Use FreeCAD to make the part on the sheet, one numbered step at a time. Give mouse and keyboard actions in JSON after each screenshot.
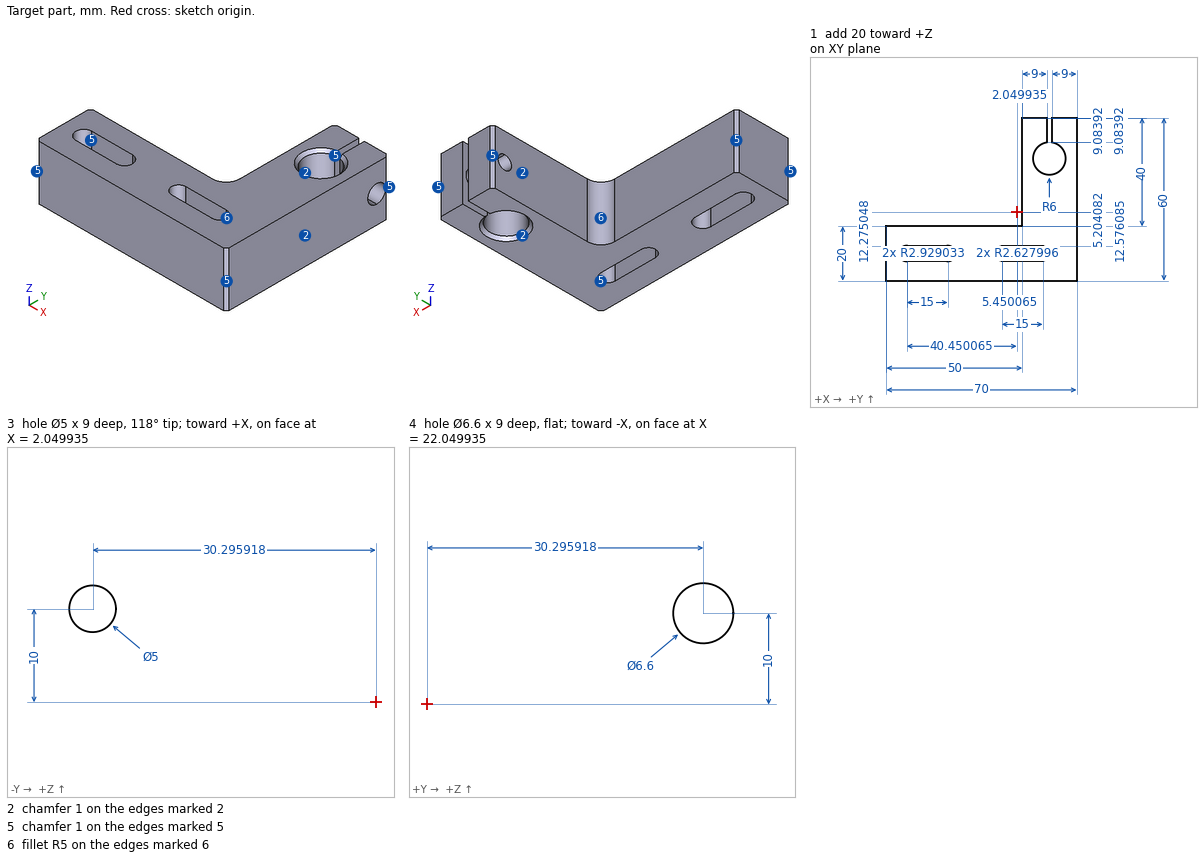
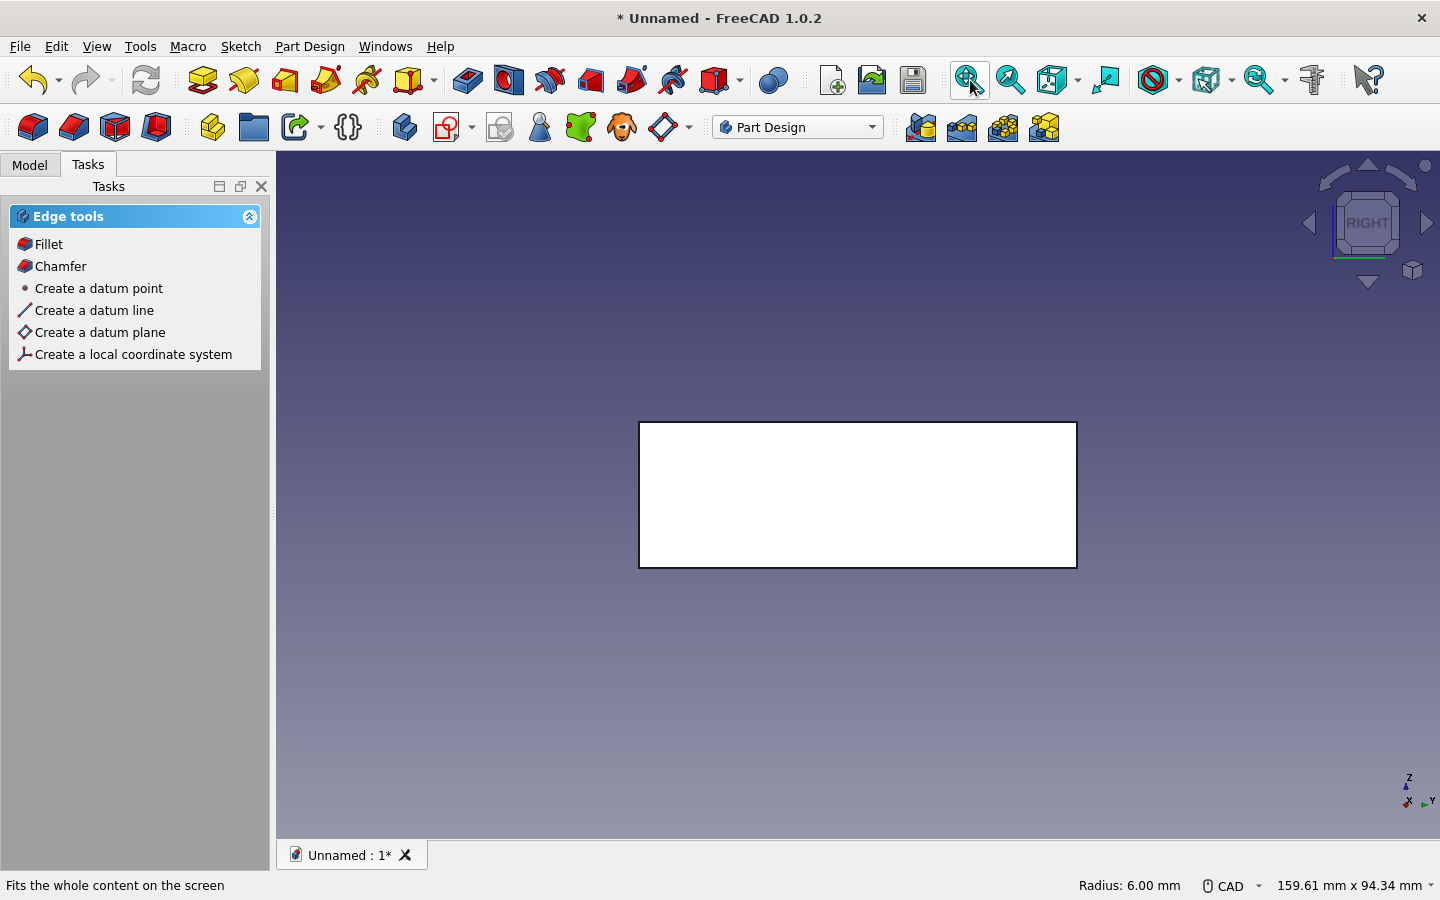
{"action": "key", "text": "5"}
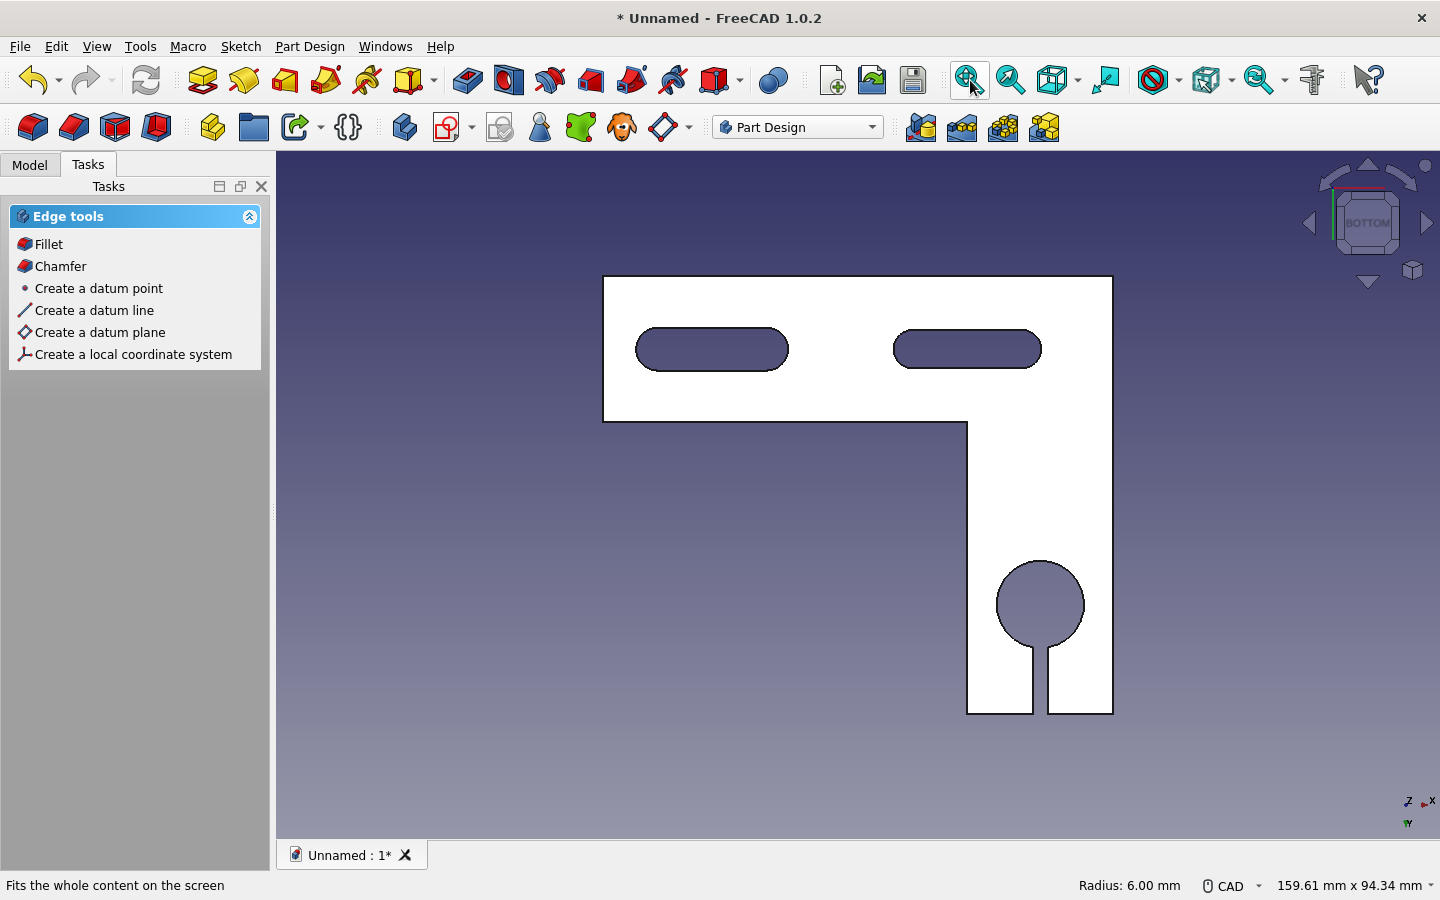
{"action": "left_click", "coordinate": [1016, 567], "text": "ctrl"}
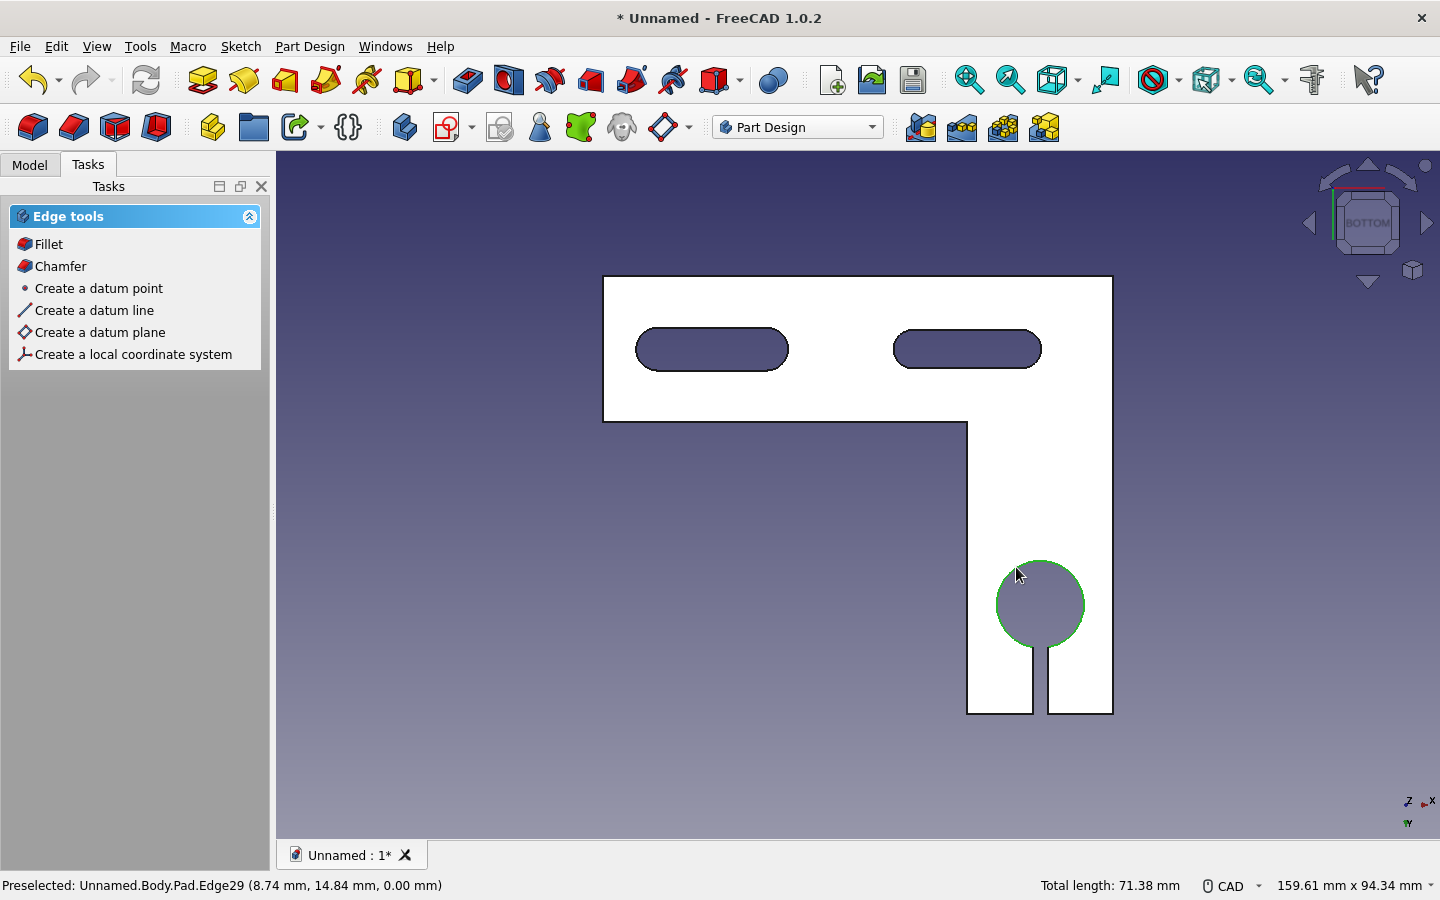
{"action": "left_click", "coordinate": [74, 128]}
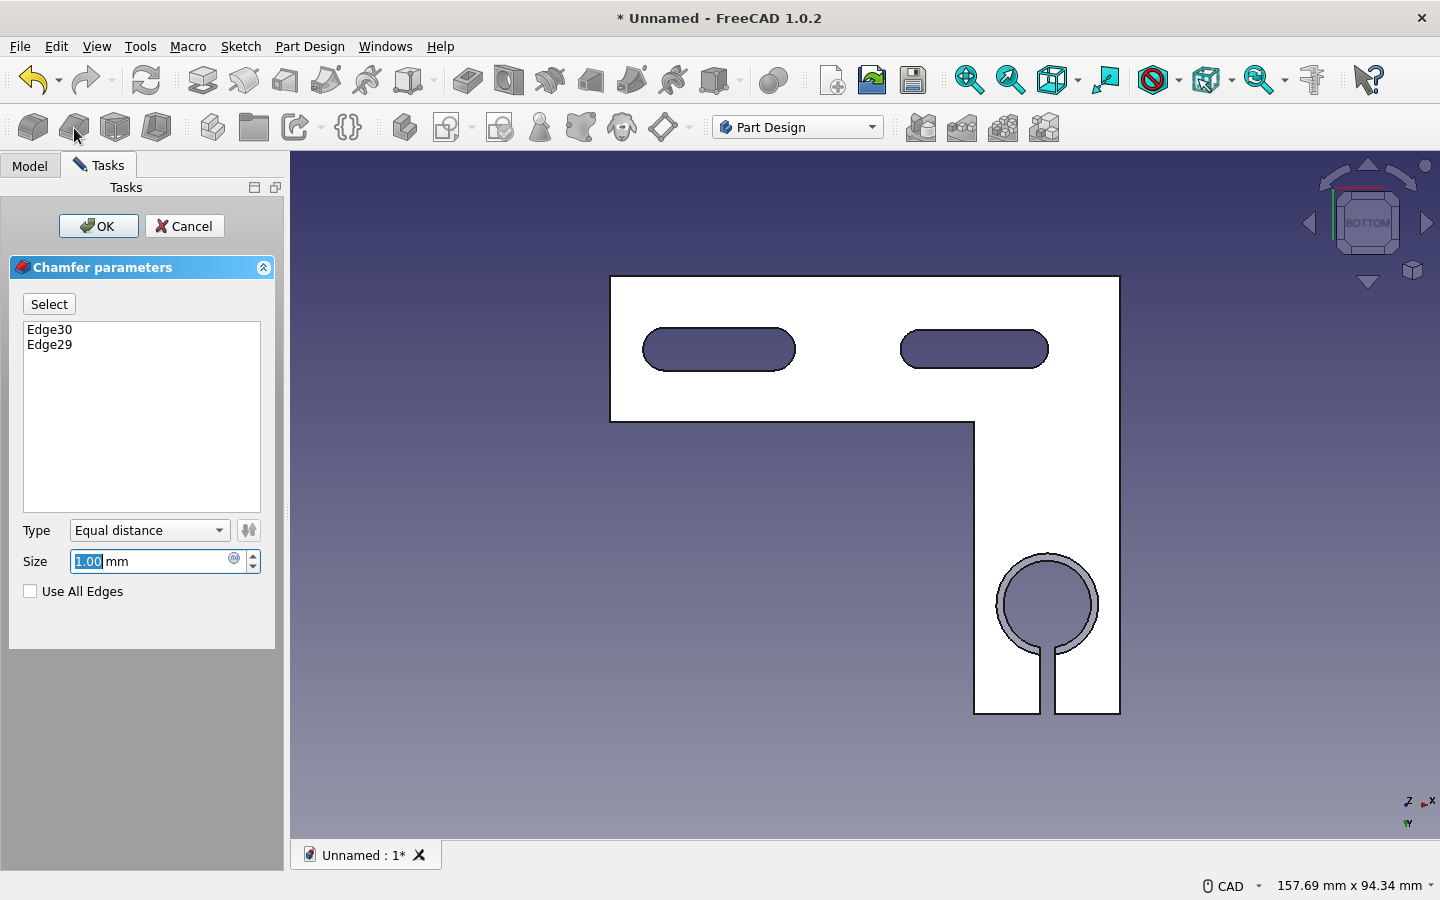
{"action": "type", "text": "1"}
{"action": "key", "text": "Tab"}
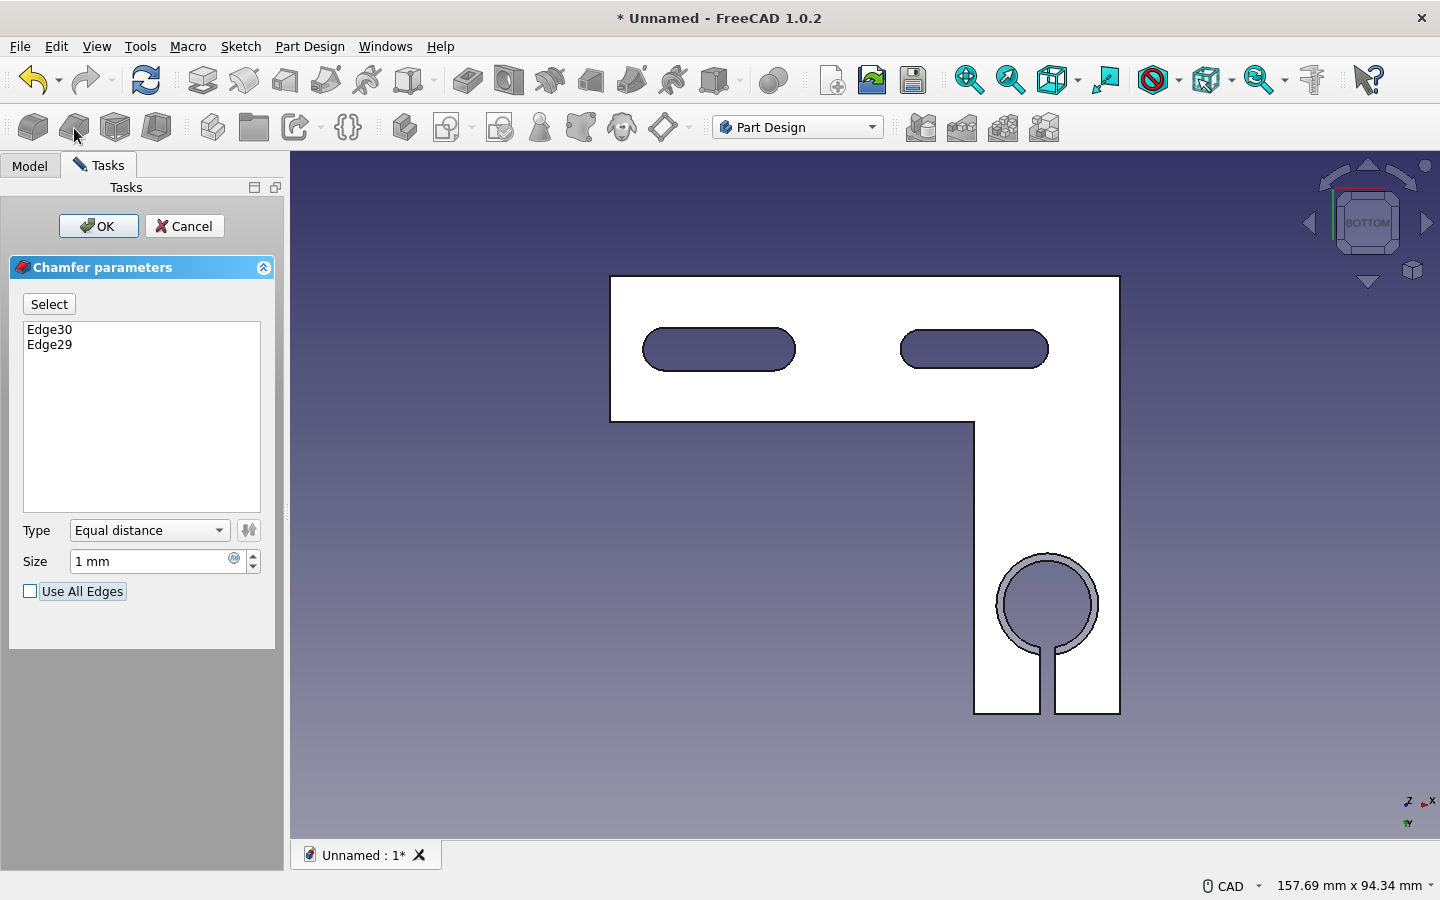
{"action": "left_click", "coordinate": [99, 226]}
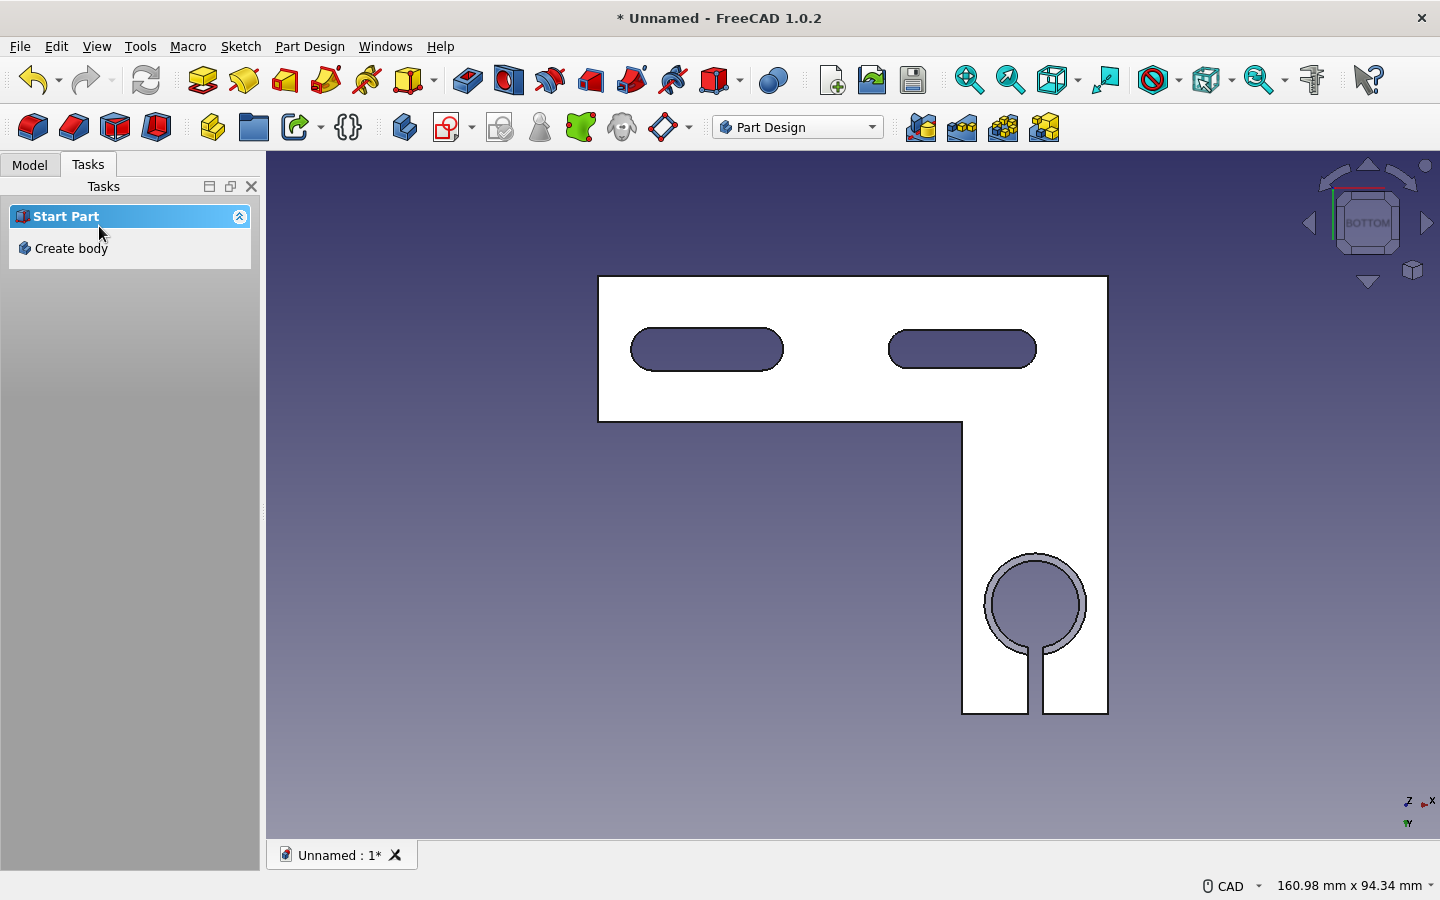
{"action": "key", "text": "6"}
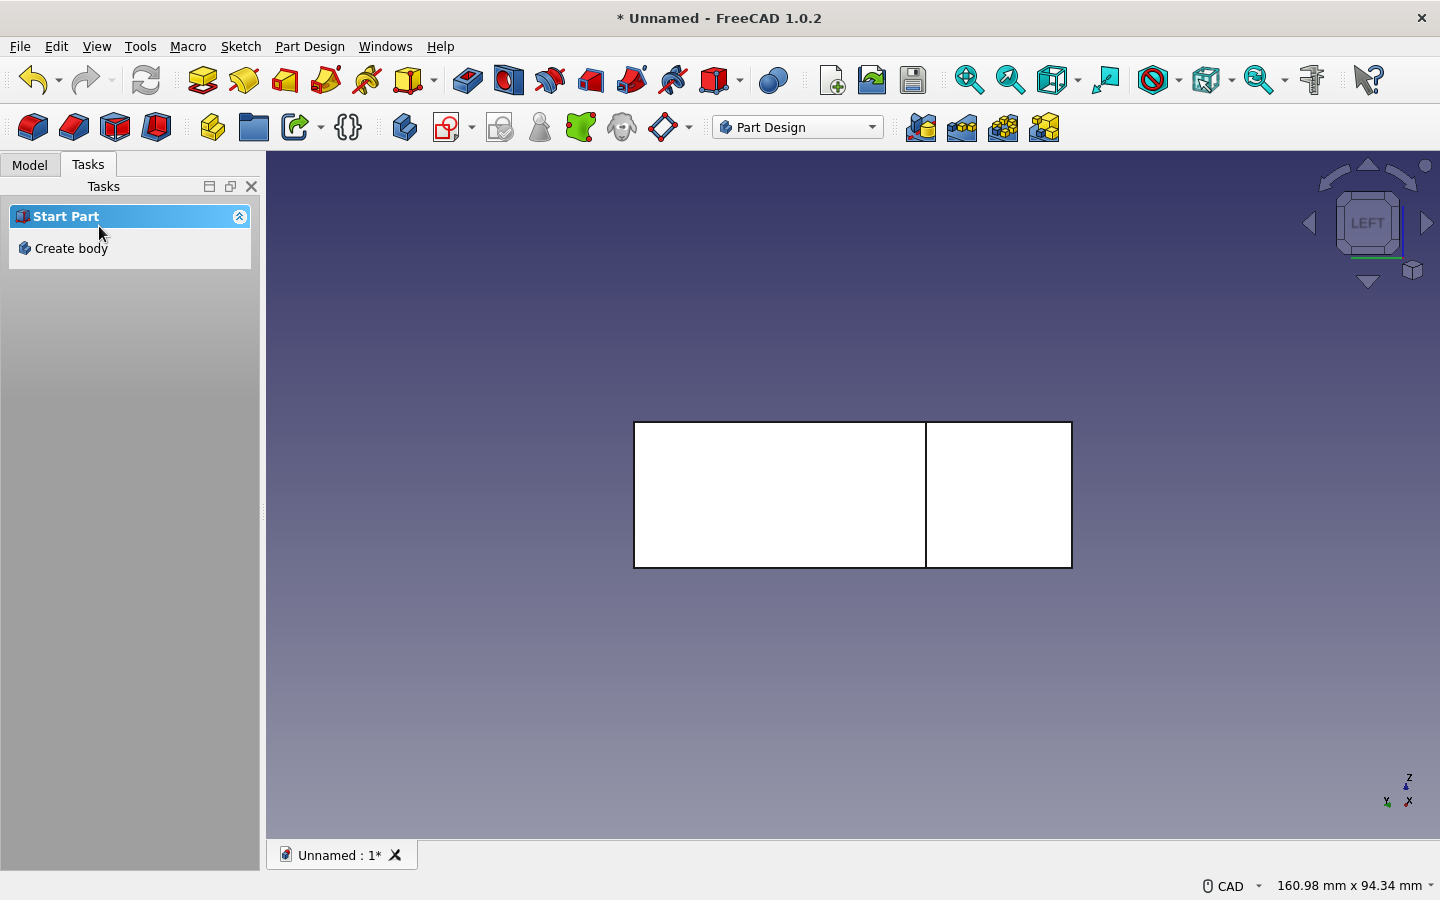
{"action": "left_click", "coordinate": [970, 80]}